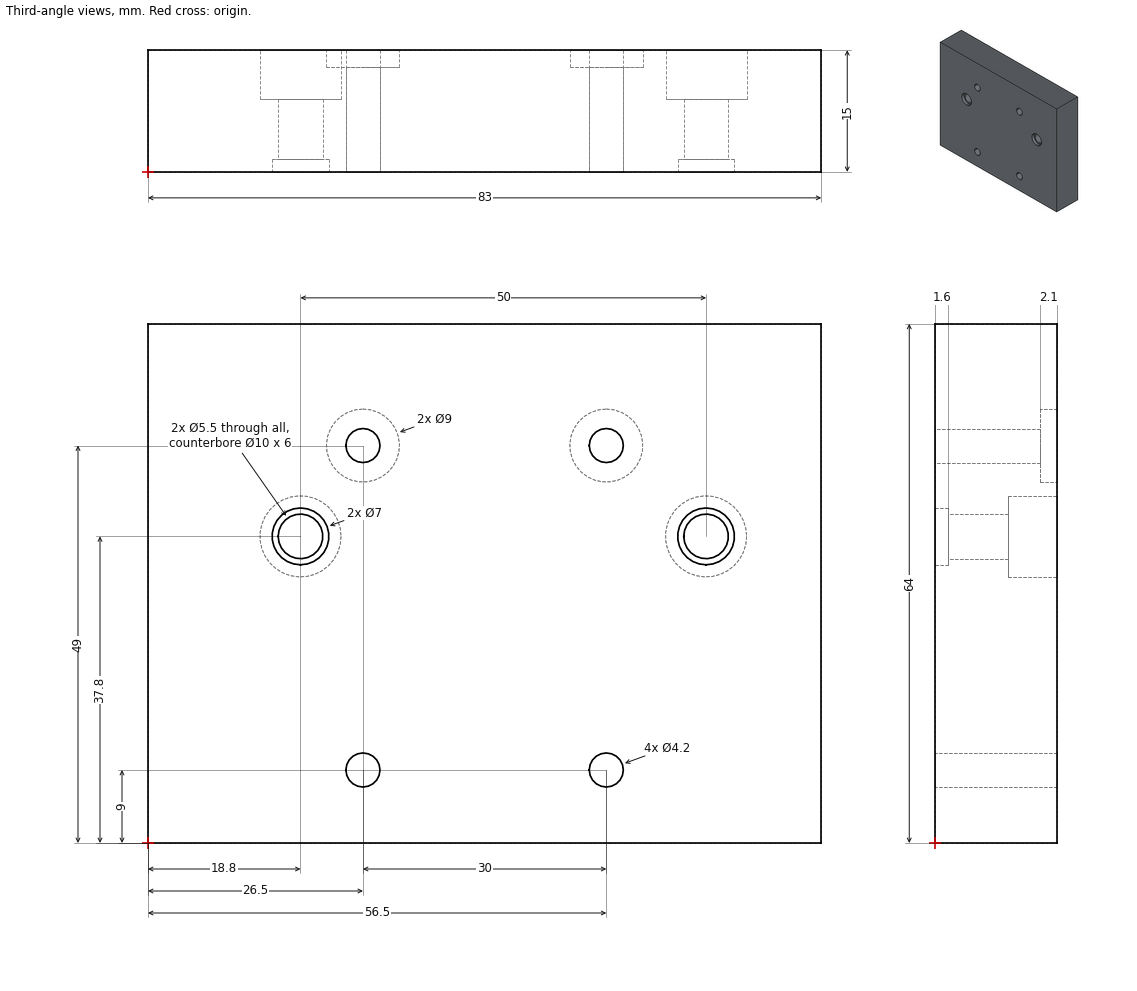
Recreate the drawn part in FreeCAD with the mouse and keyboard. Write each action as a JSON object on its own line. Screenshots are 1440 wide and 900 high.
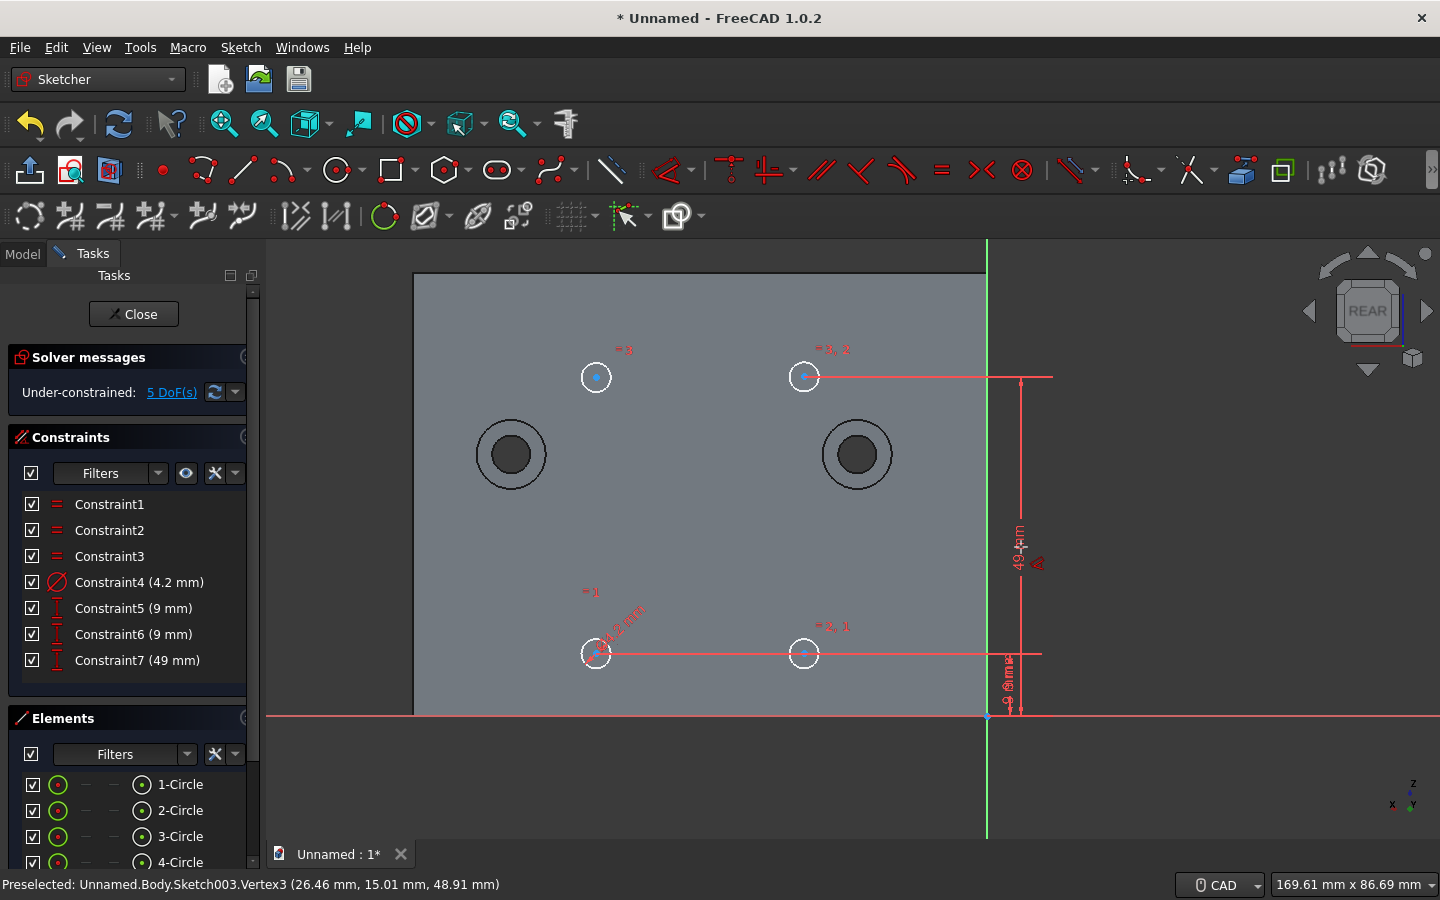
{"action": "left_click", "coordinate": [596, 378]}
{"action": "left_click", "coordinate": [1021, 469]}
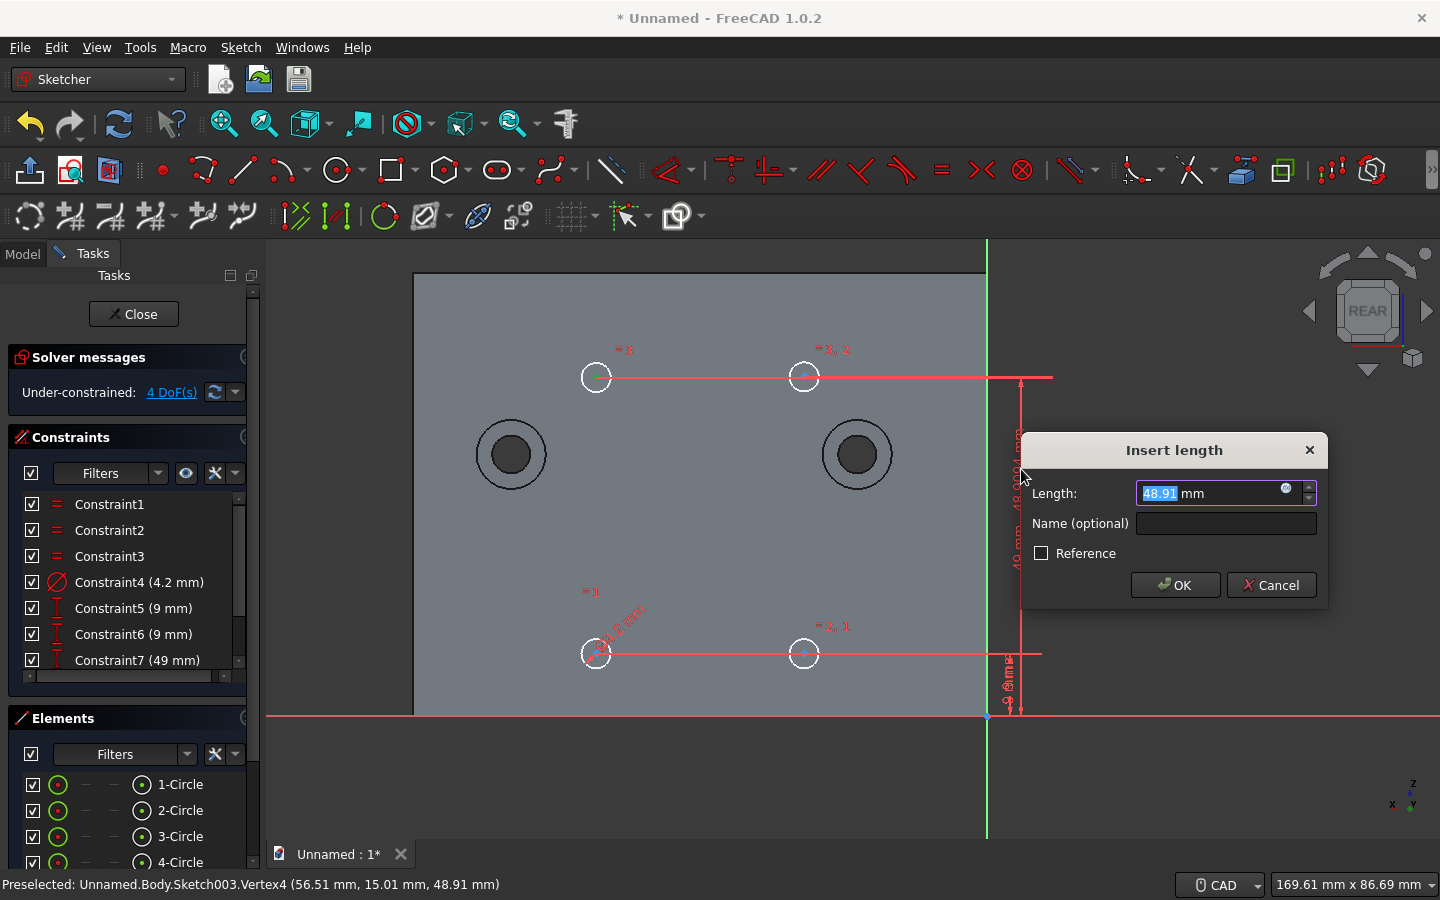
{"action": "type", "text": "49"}
{"action": "key", "text": "Return"}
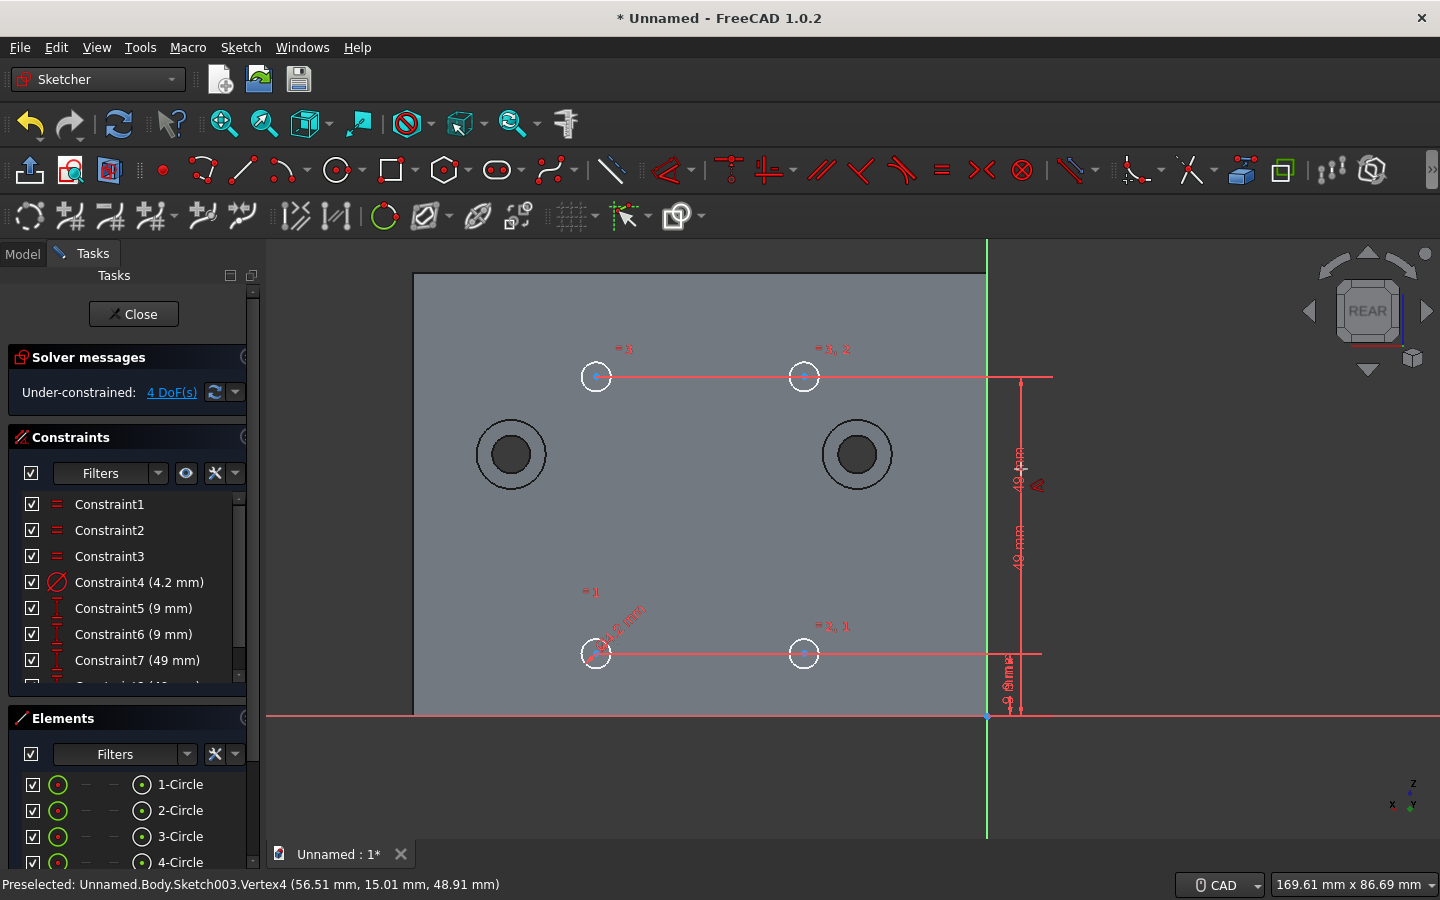
{"action": "left_click", "coordinate": [596, 654]}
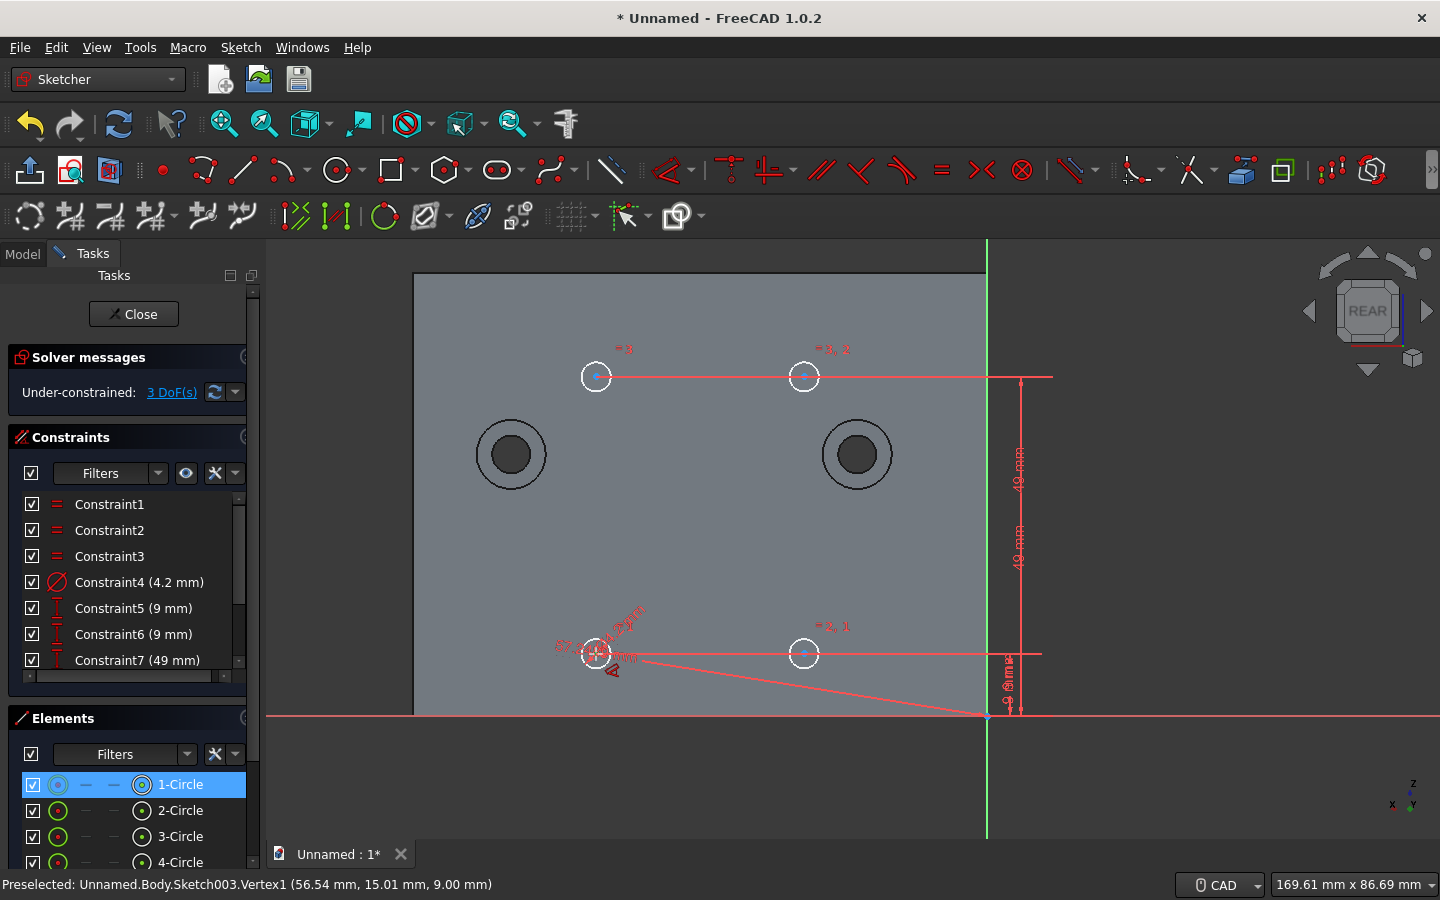
{"action": "left_click", "coordinate": [804, 654]}
{"action": "left_click", "coordinate": [700, 688]}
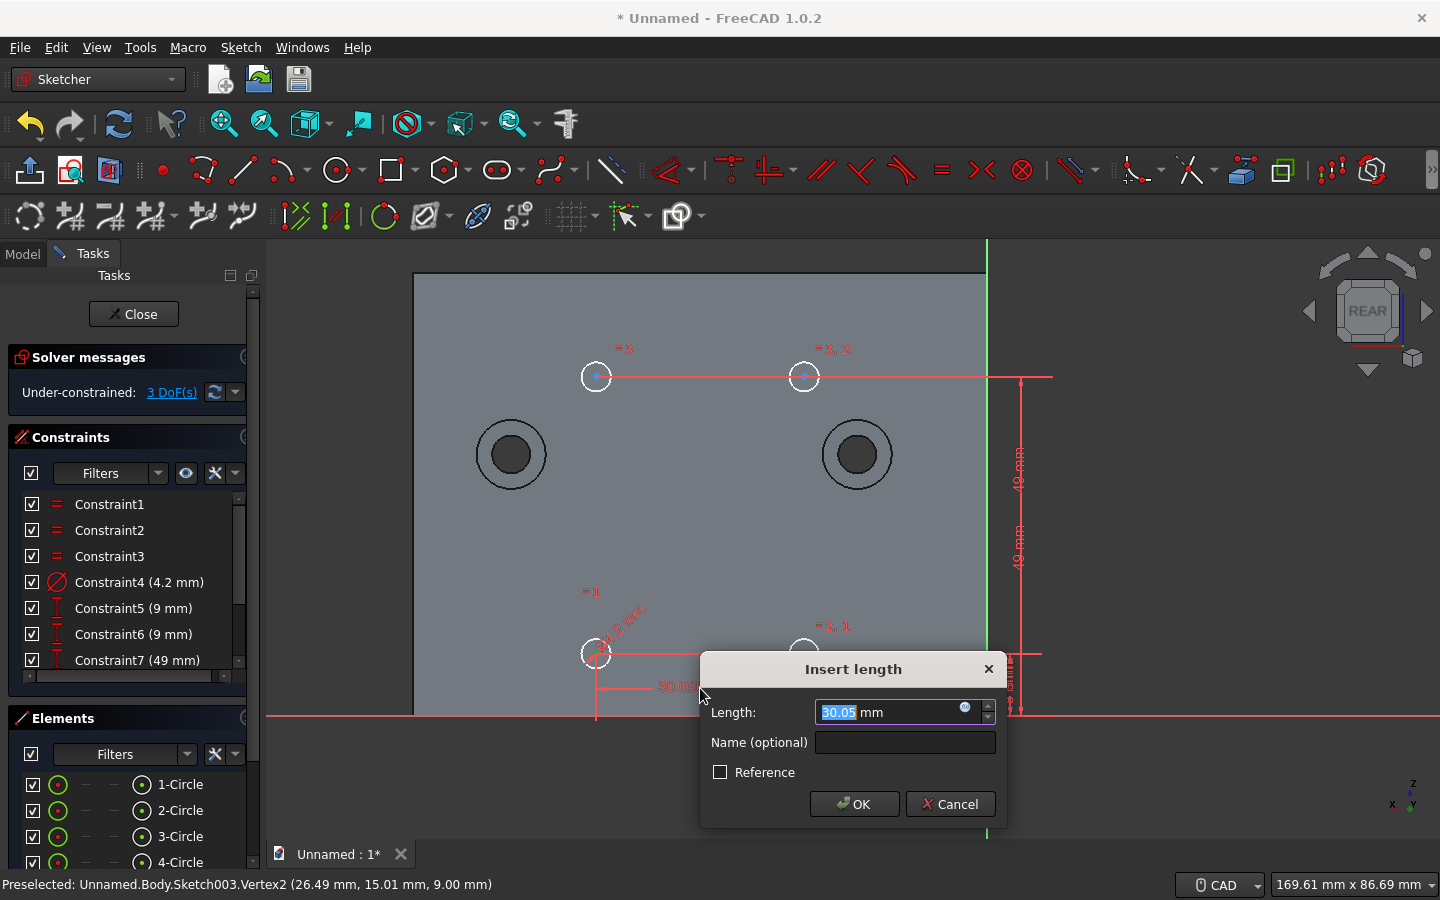
{"action": "type", "text": "30"}
{"action": "key", "text": "Return"}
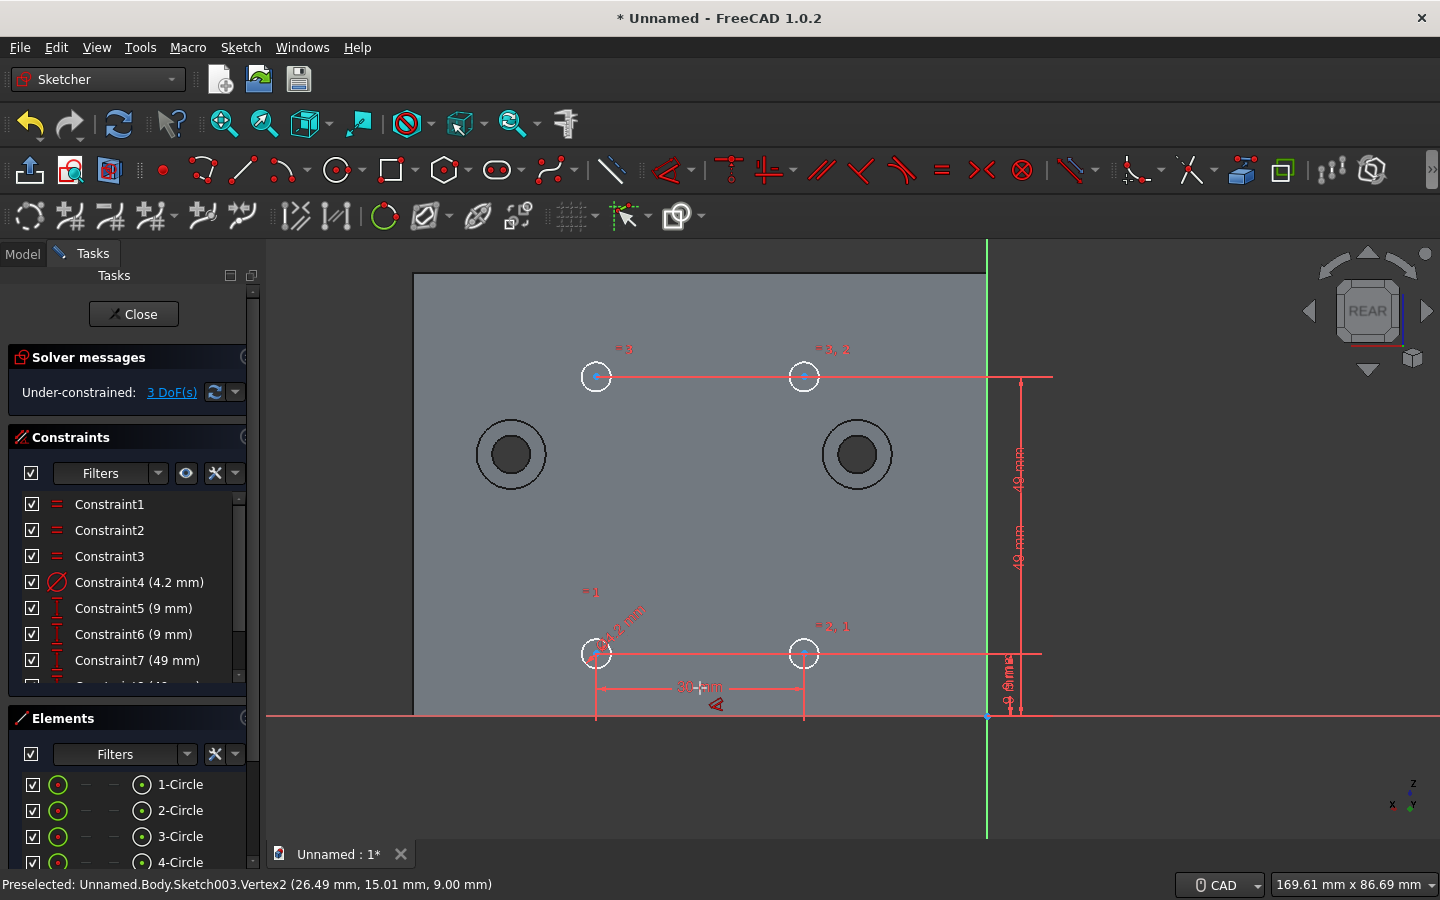
{"action": "left_click", "coordinate": [596, 654]}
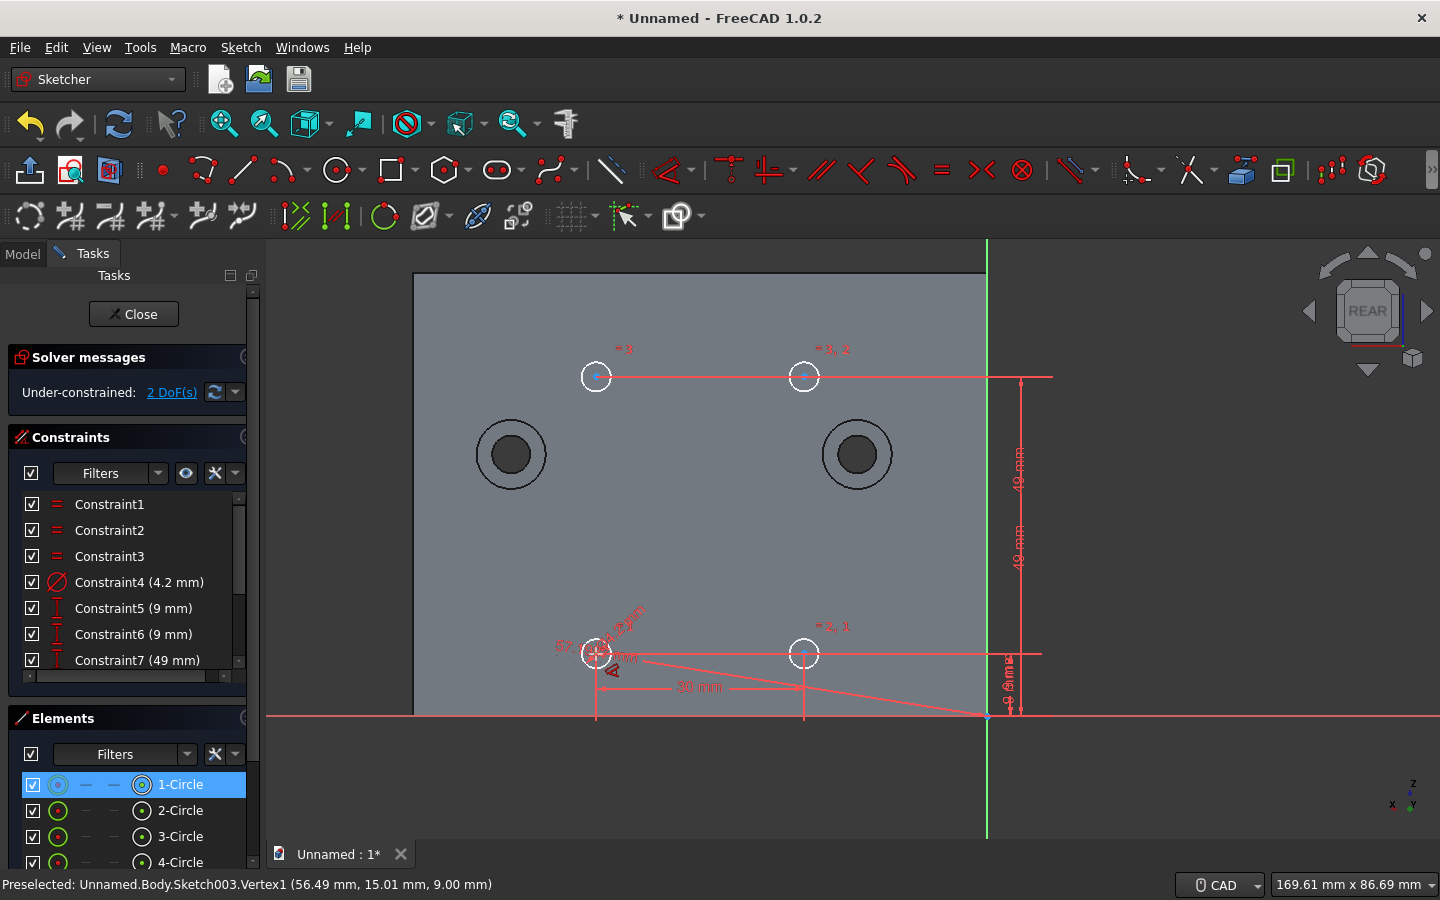
{"action": "left_click", "coordinate": [804, 377]}
{"action": "left_click", "coordinate": [700, 343]}